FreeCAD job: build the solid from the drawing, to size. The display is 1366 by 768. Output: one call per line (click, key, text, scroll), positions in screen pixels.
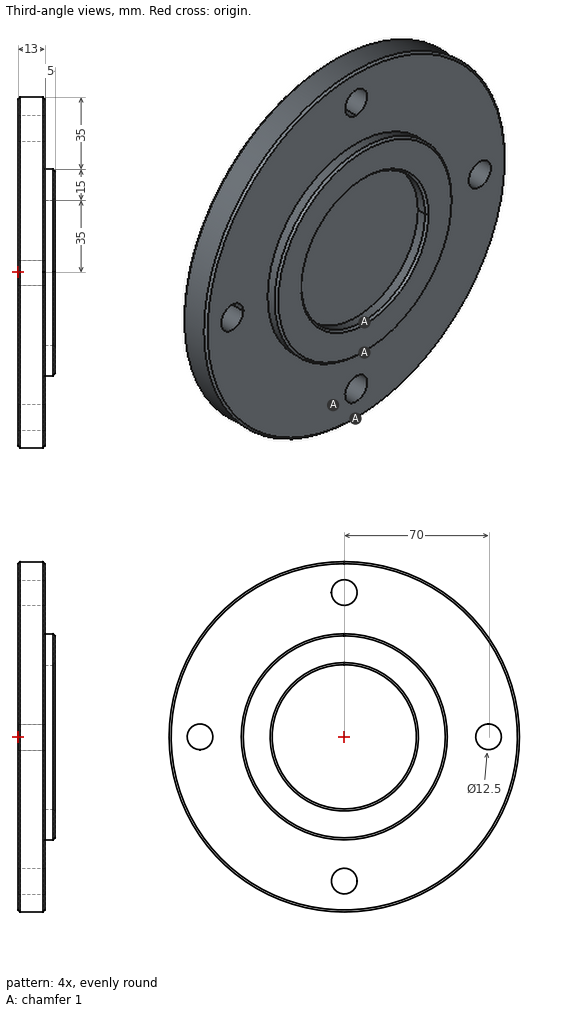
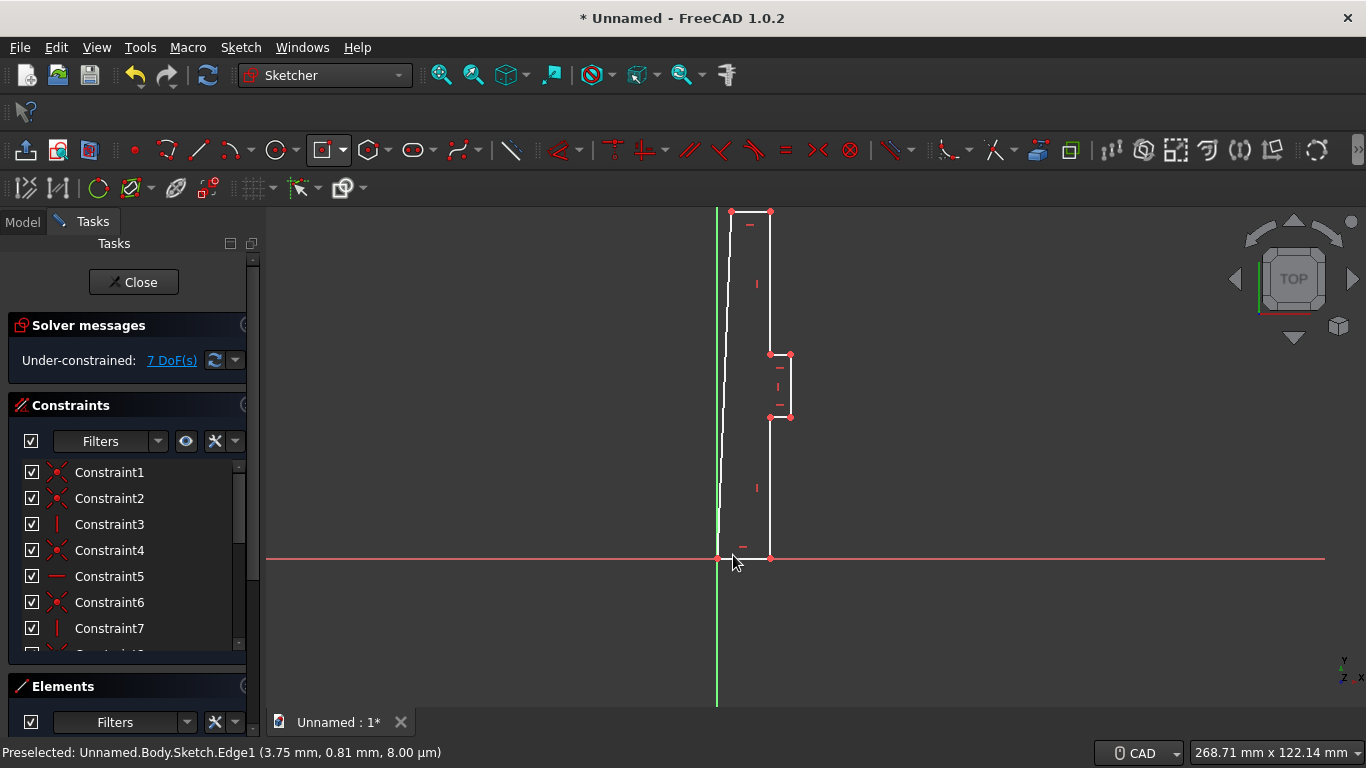
scroll(727, 316, up, 2)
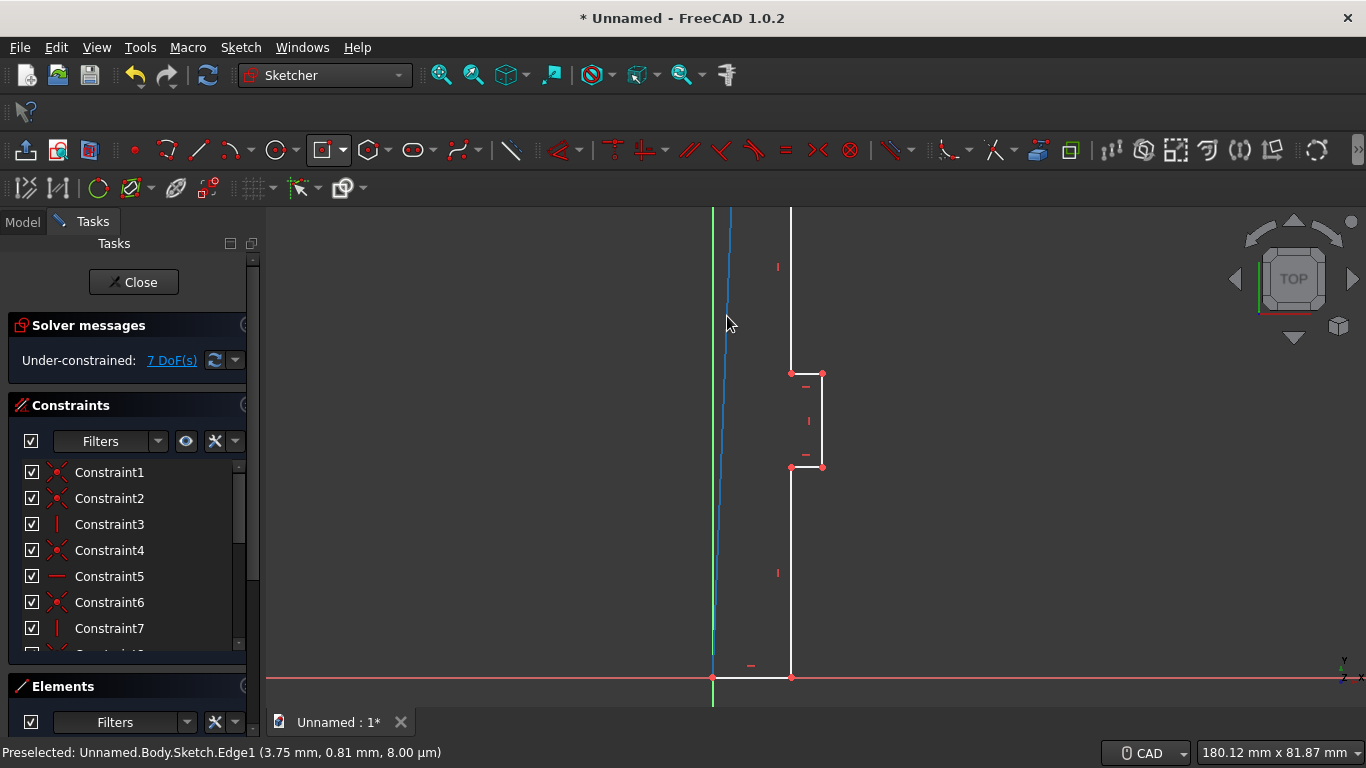
click(727, 315)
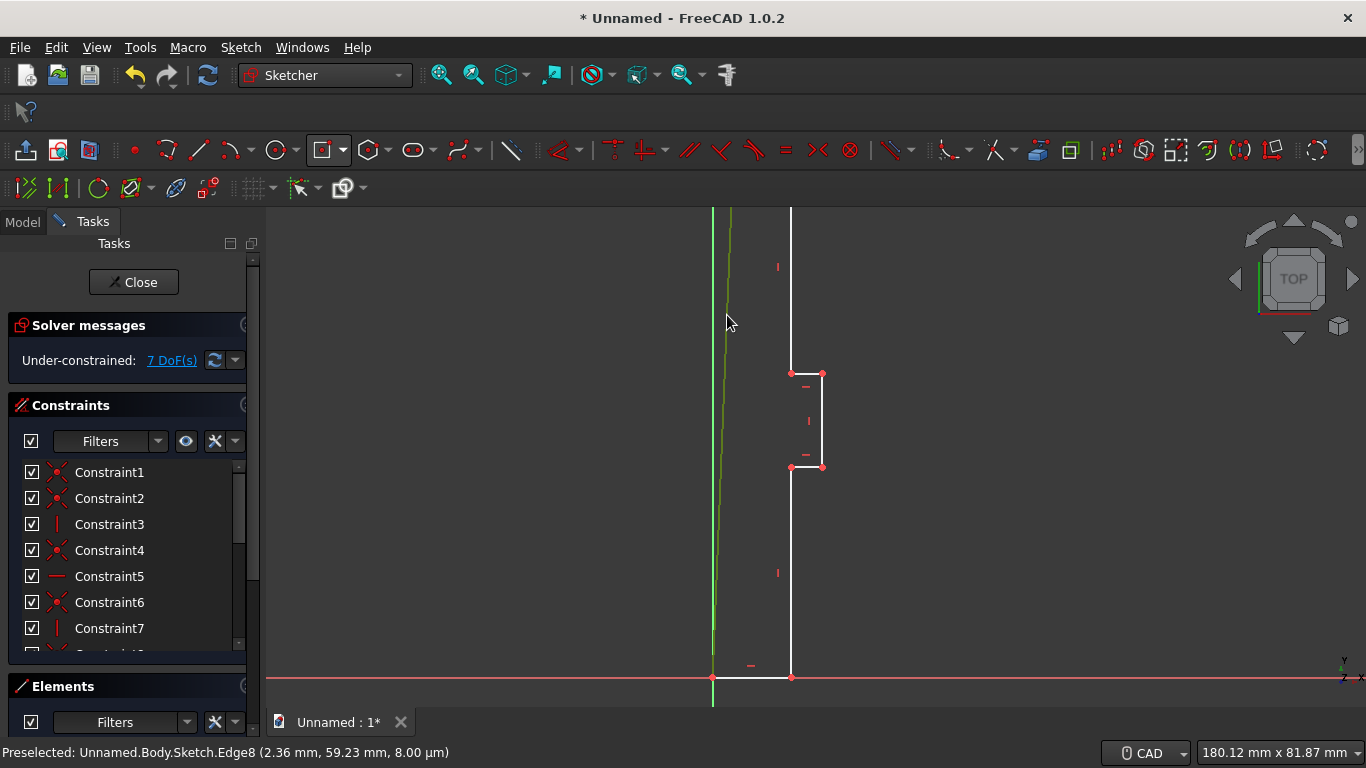
key(v)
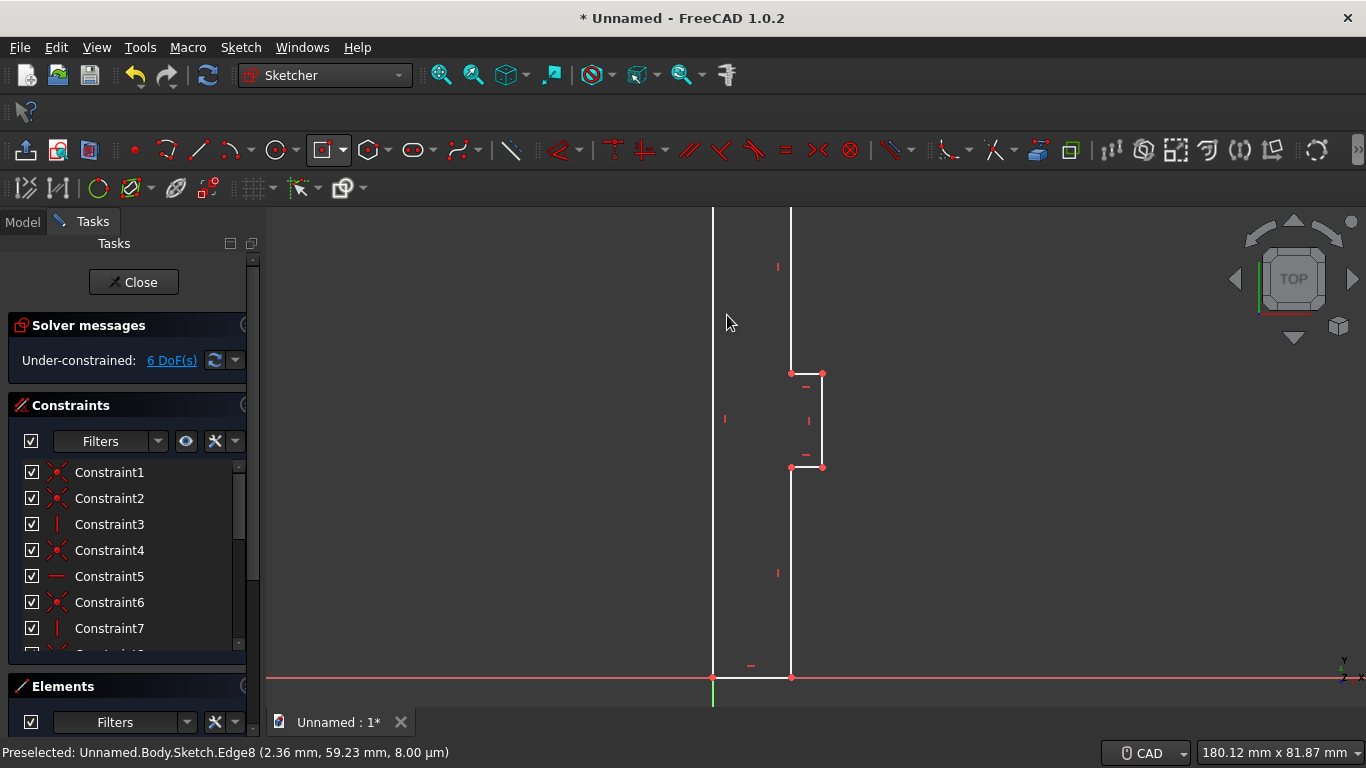
click(558, 150)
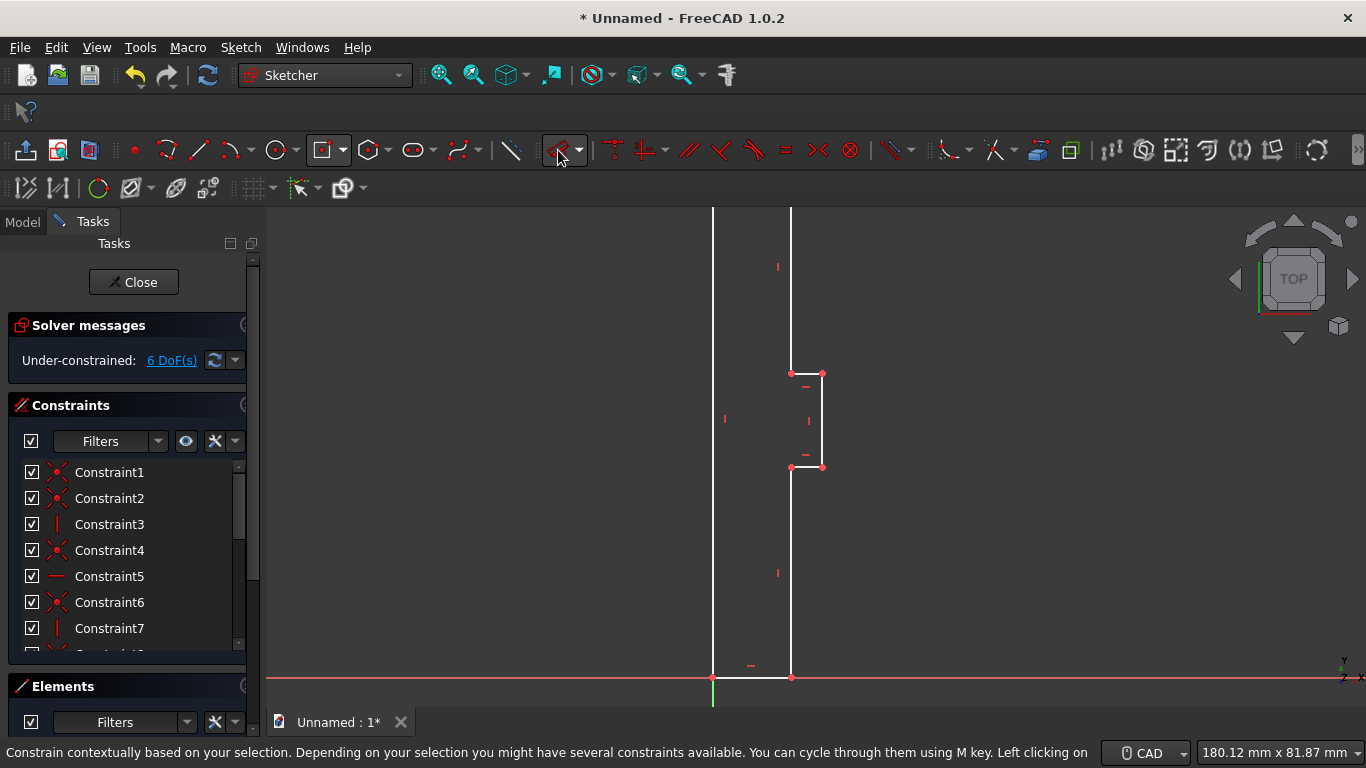
scroll(800, 467, up, 2)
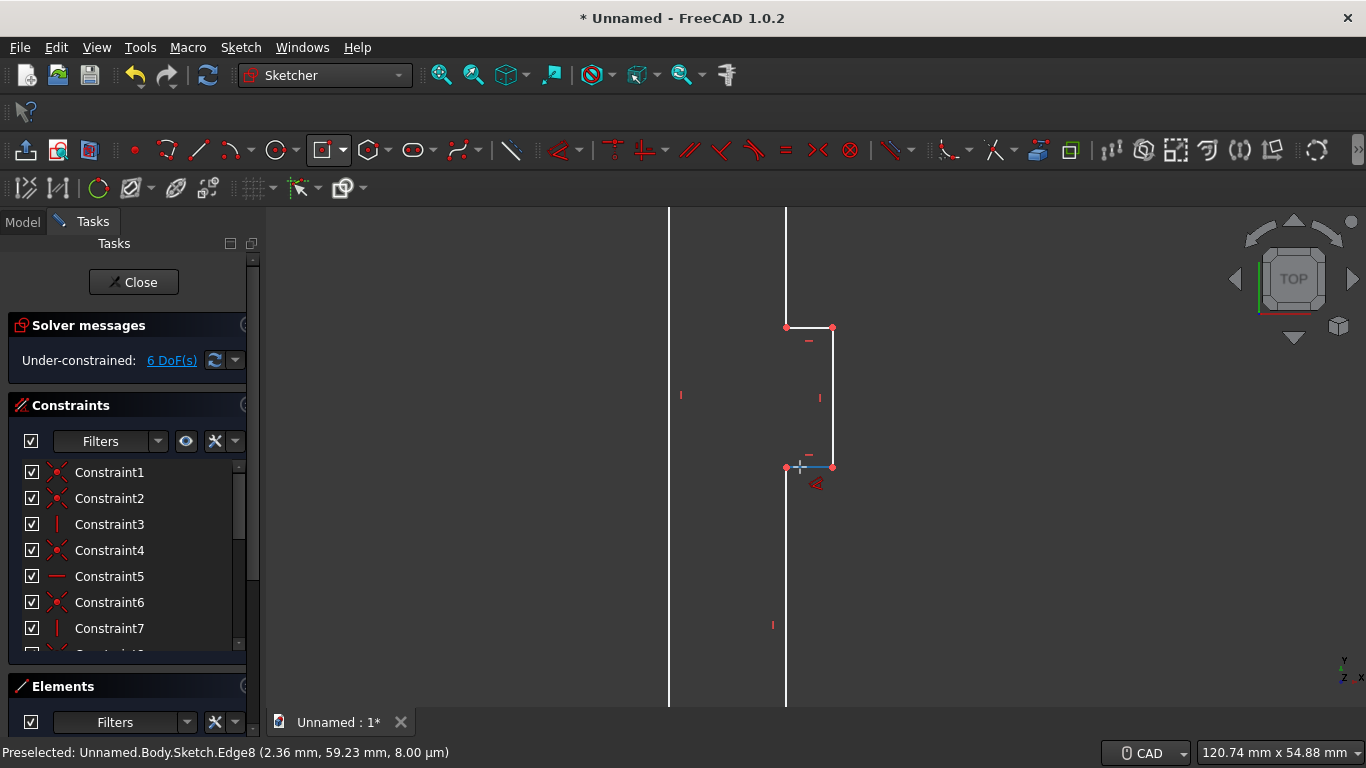
click(800, 467)
click(810, 501)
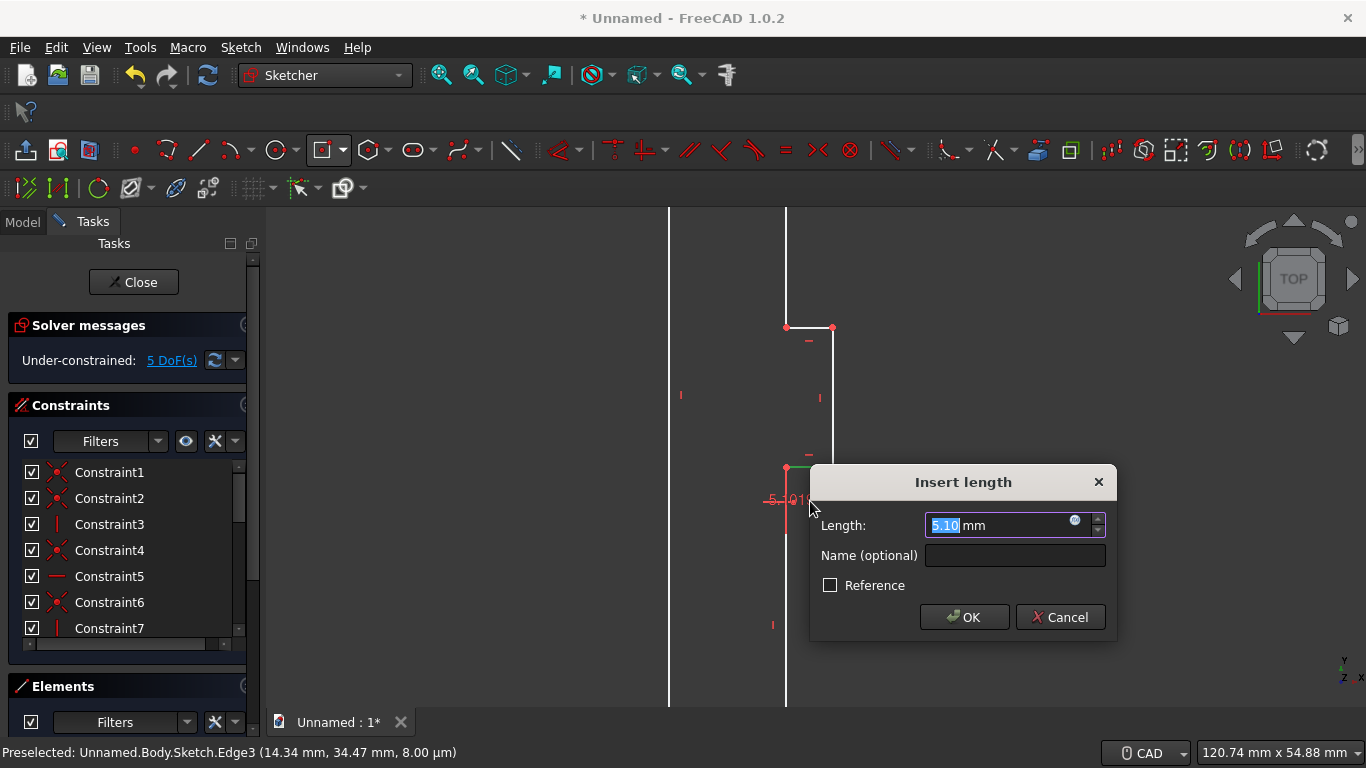
text(5)
key(Return)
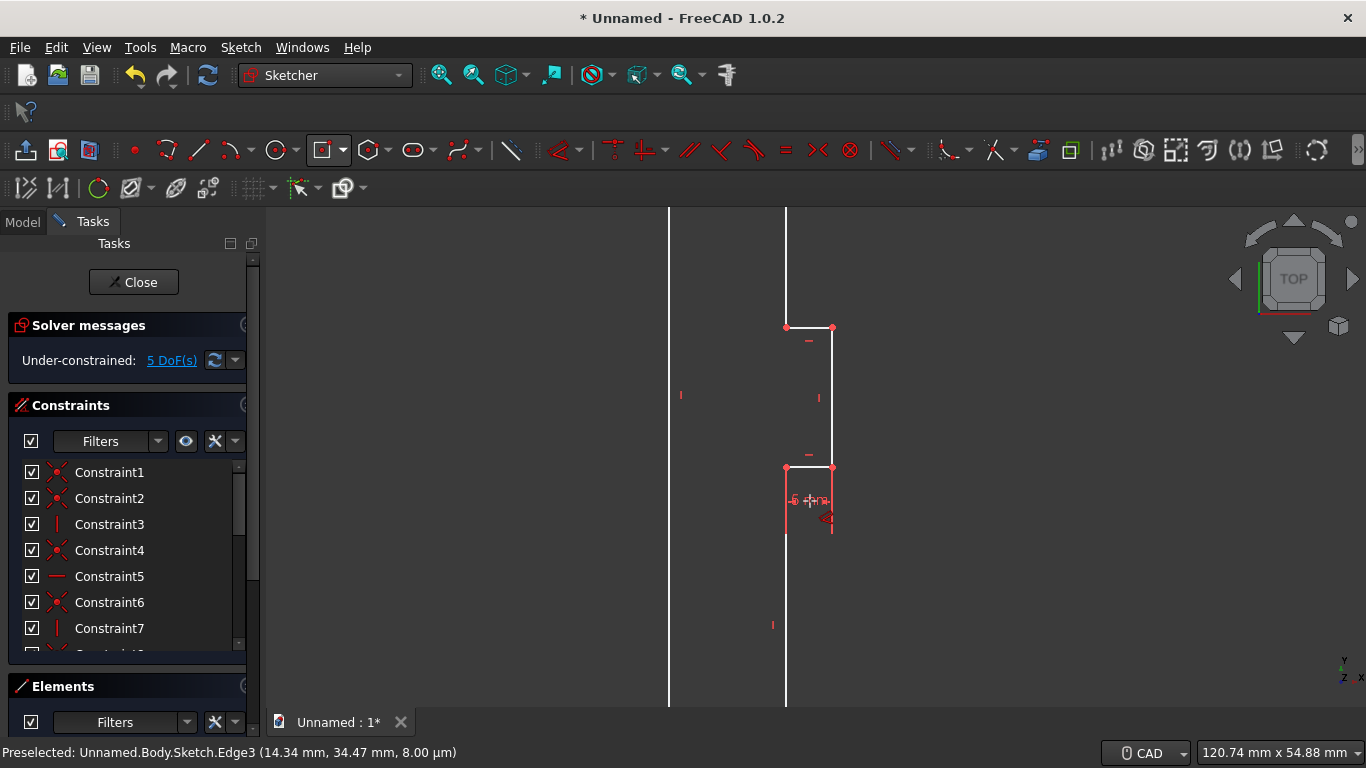
click(818, 328)
click(809, 294)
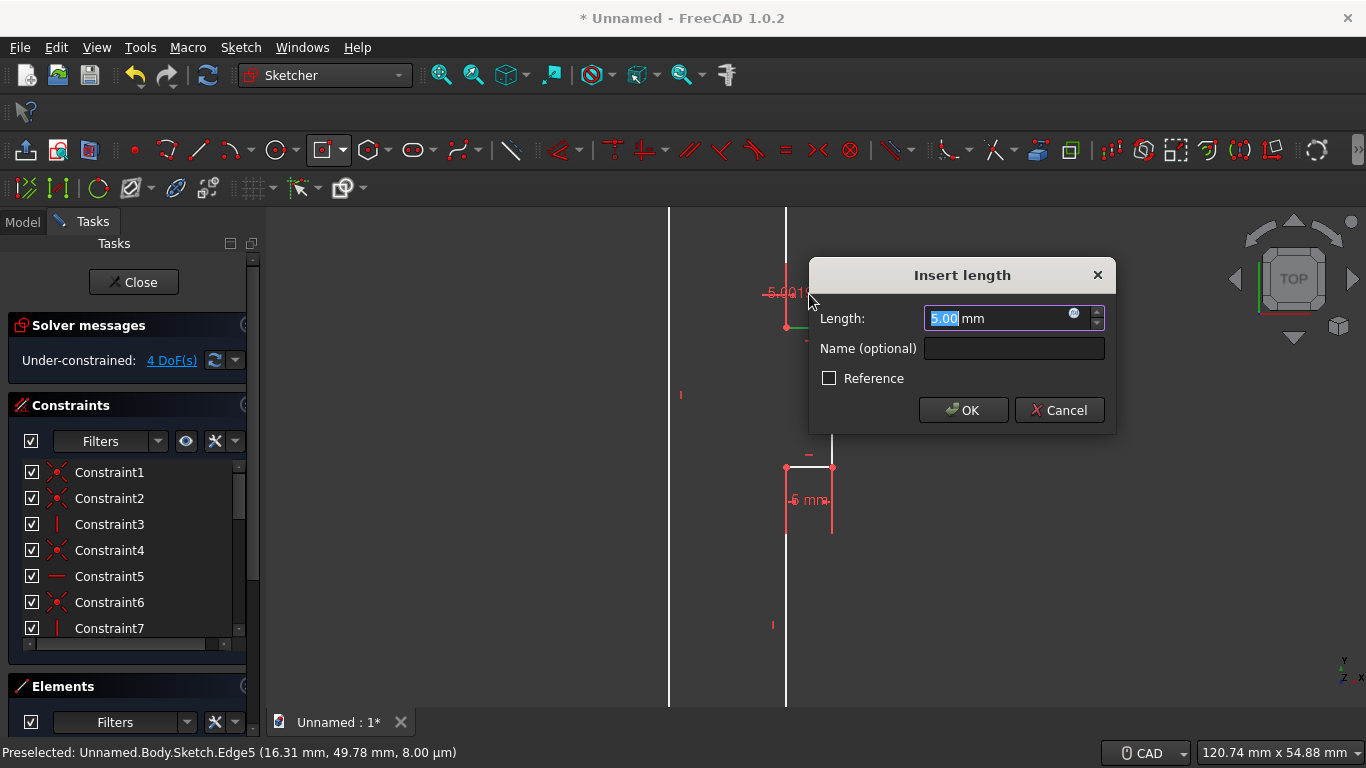
text(5)
key(Return)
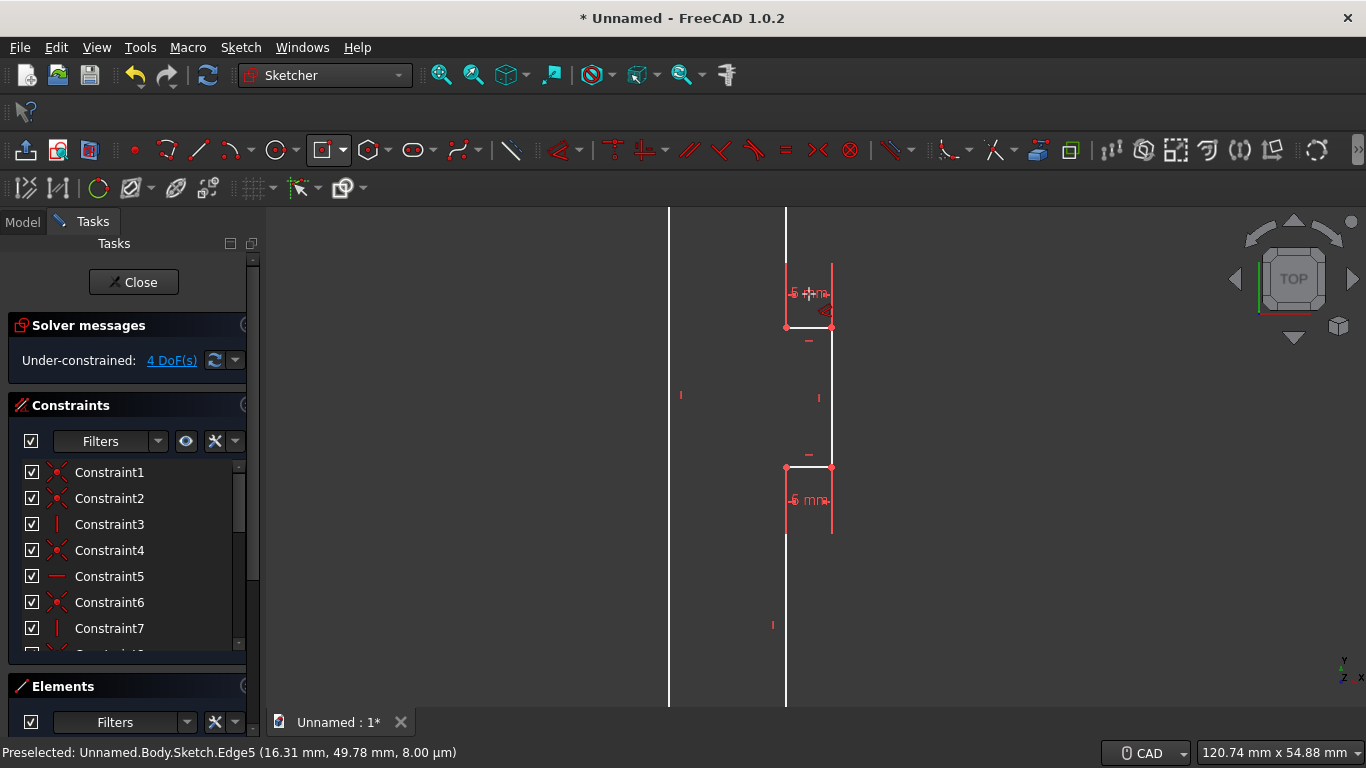
scroll(745, 494, down, 5)